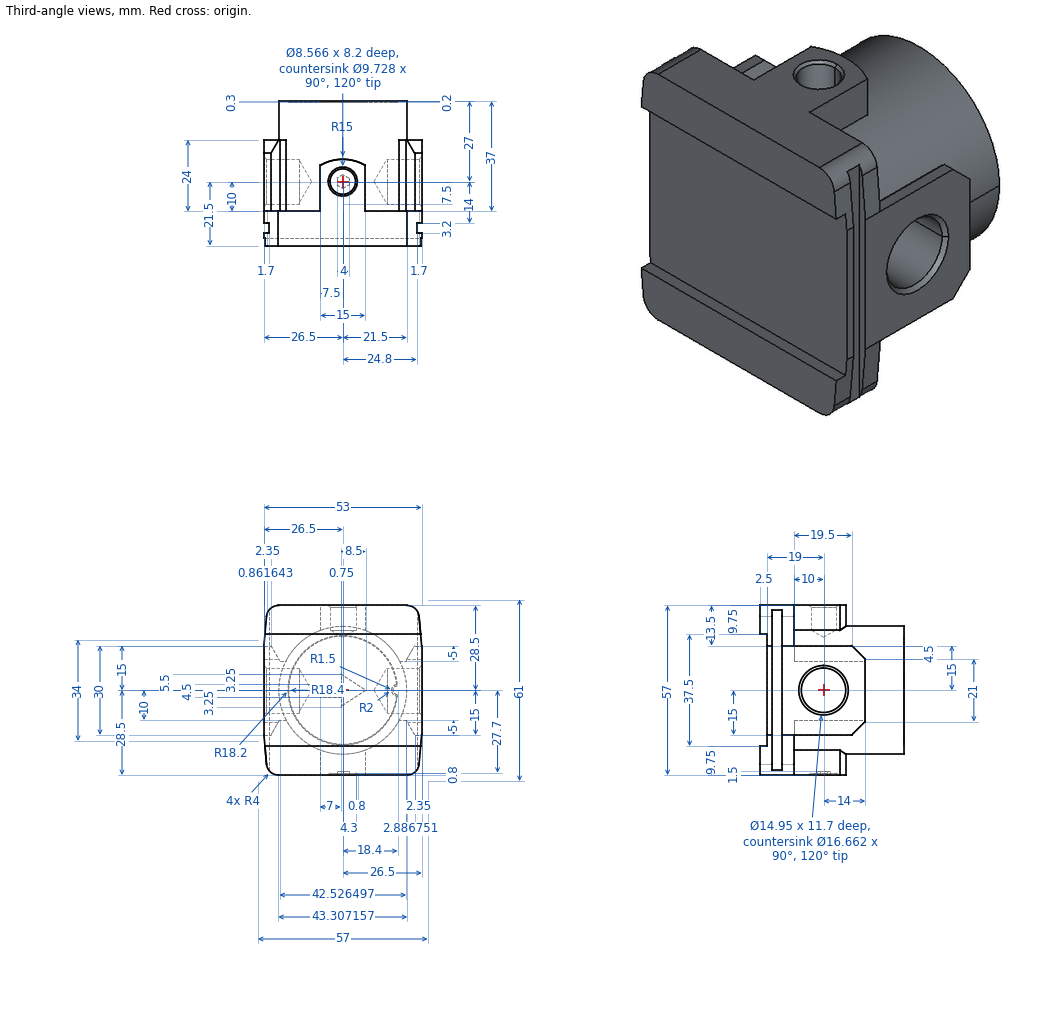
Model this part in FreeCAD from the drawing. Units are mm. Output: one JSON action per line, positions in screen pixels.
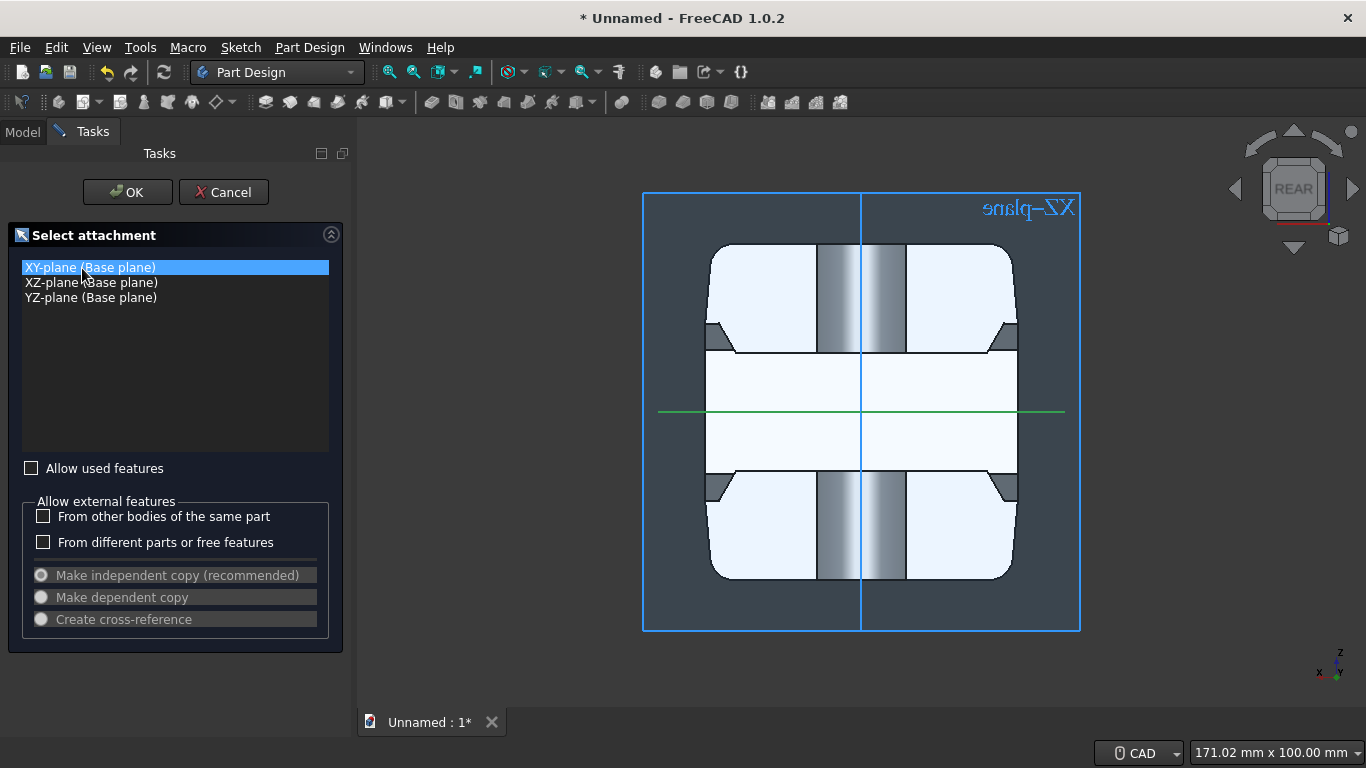
{"action": "left_click", "coordinate": [128, 192]}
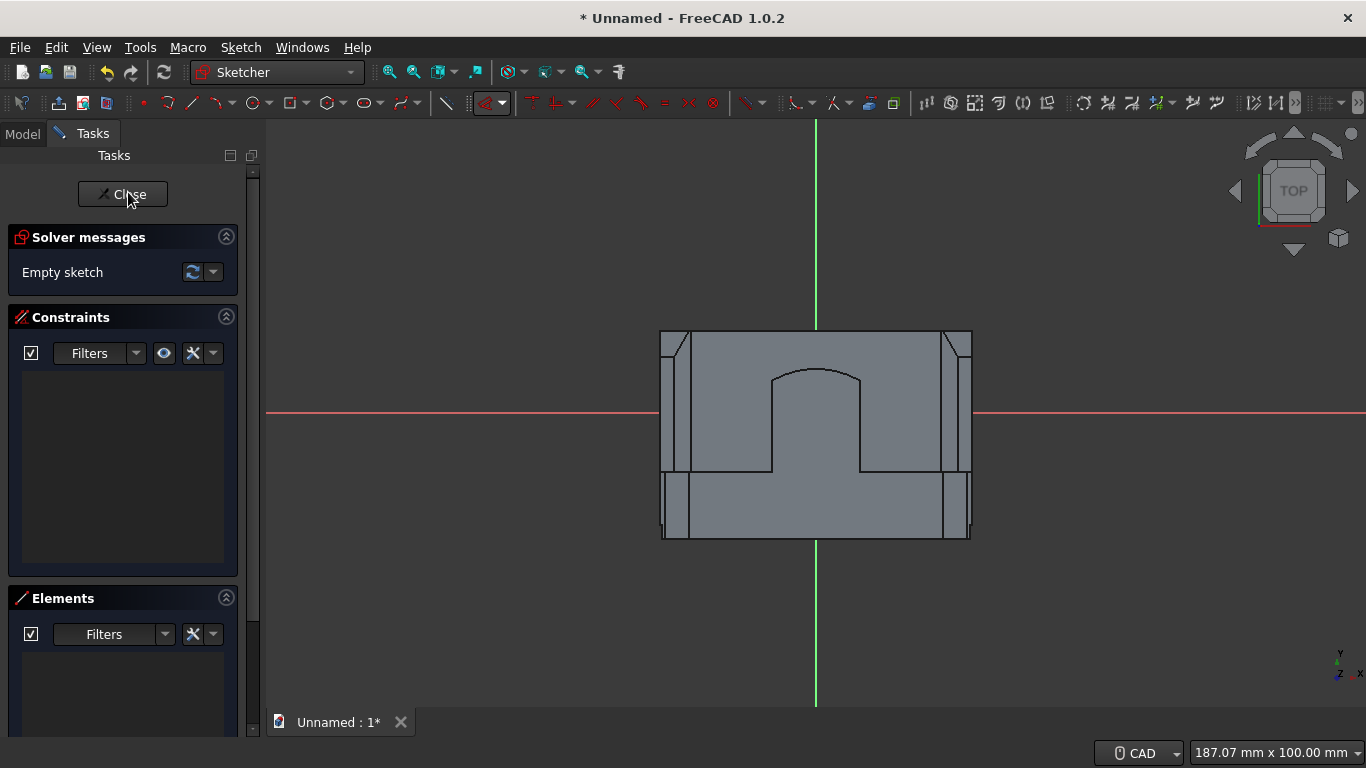
{"action": "left_click", "coordinate": [108, 104]}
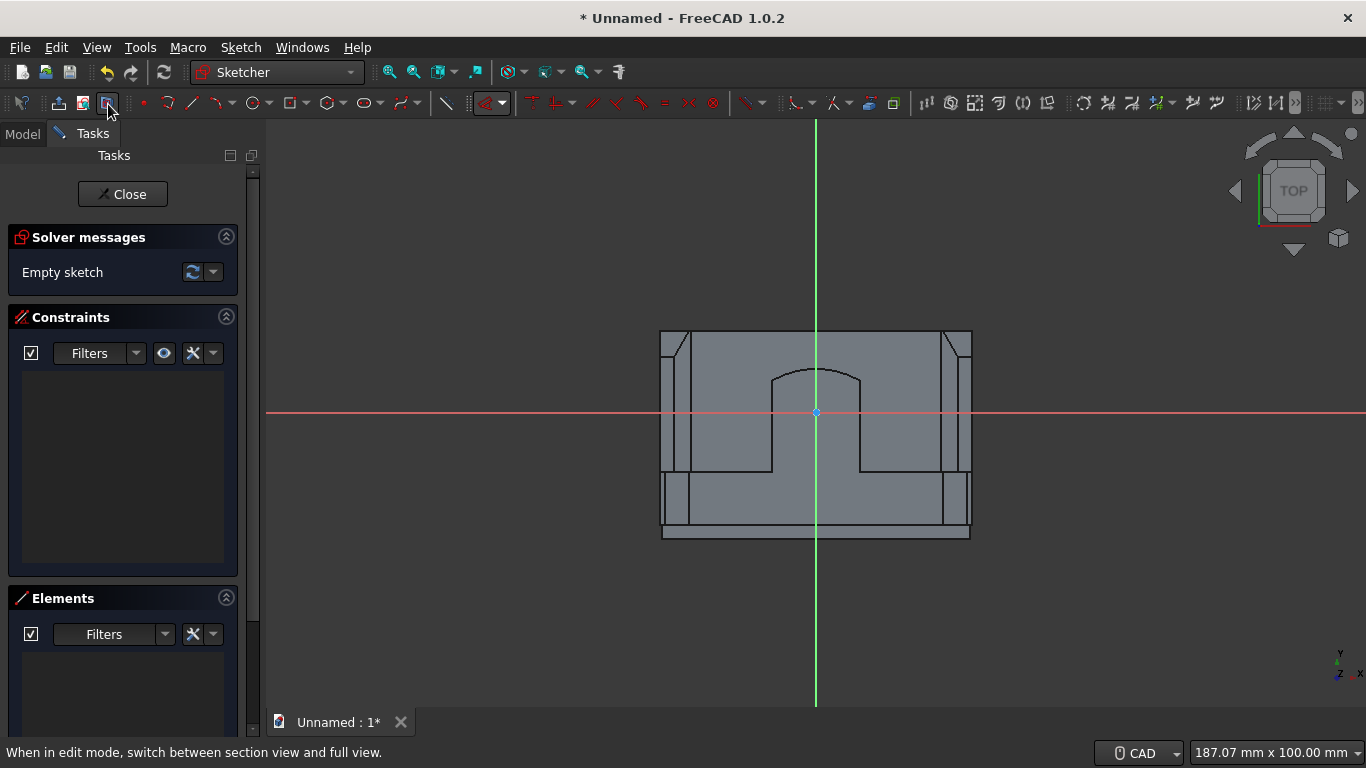
{"action": "scroll", "coordinate": [1039, 302], "scroll_direction": "up", "scroll_amount": 3}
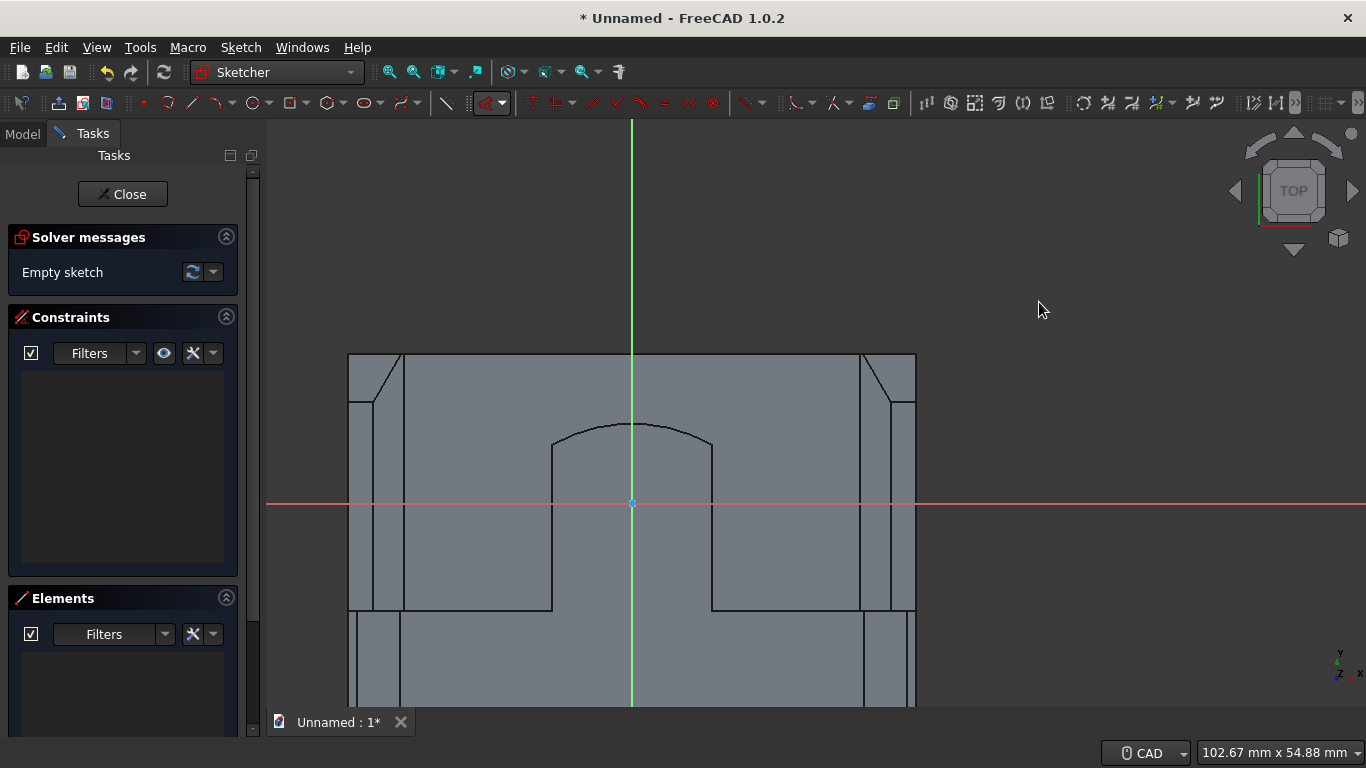
{"action": "key", "text": "g r"}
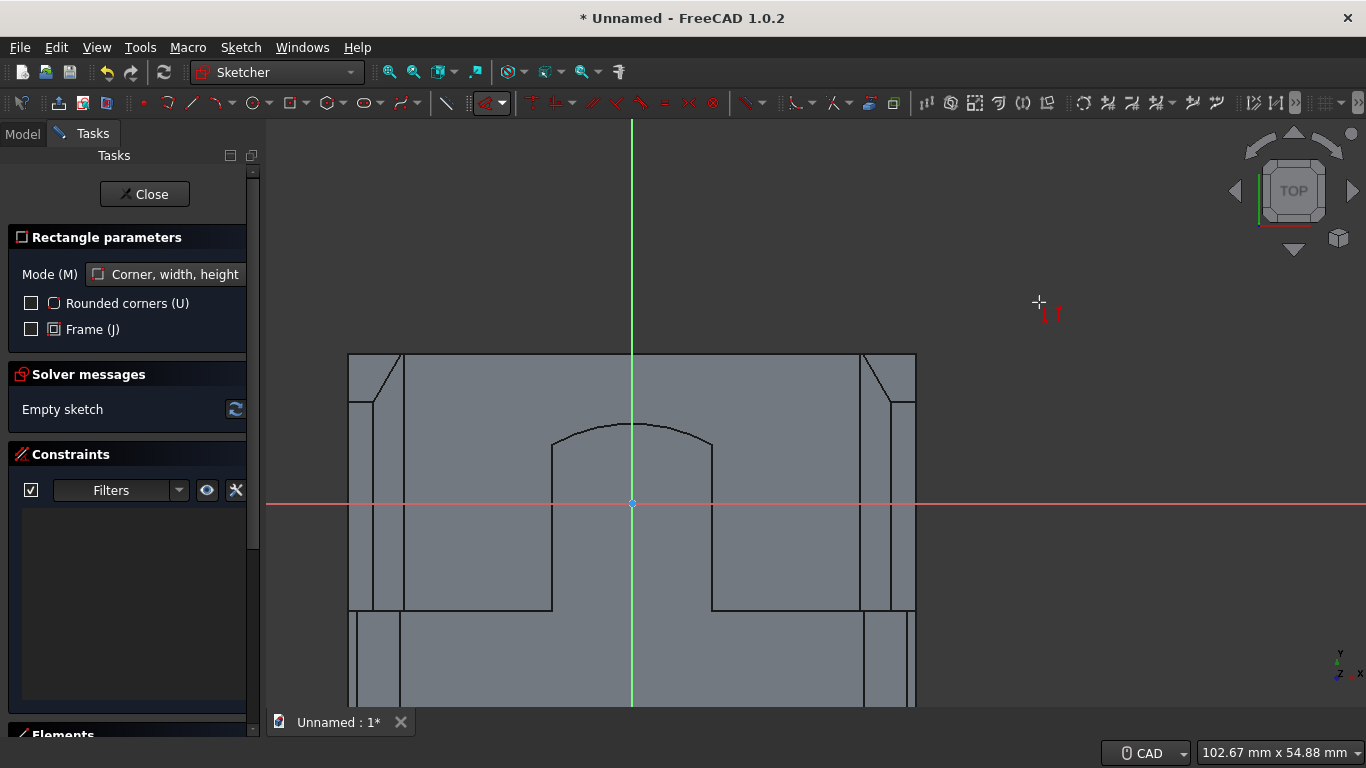
{"action": "left_click", "coordinate": [632, 215]}
{"action": "mouse_move", "coordinate": [862, 611]}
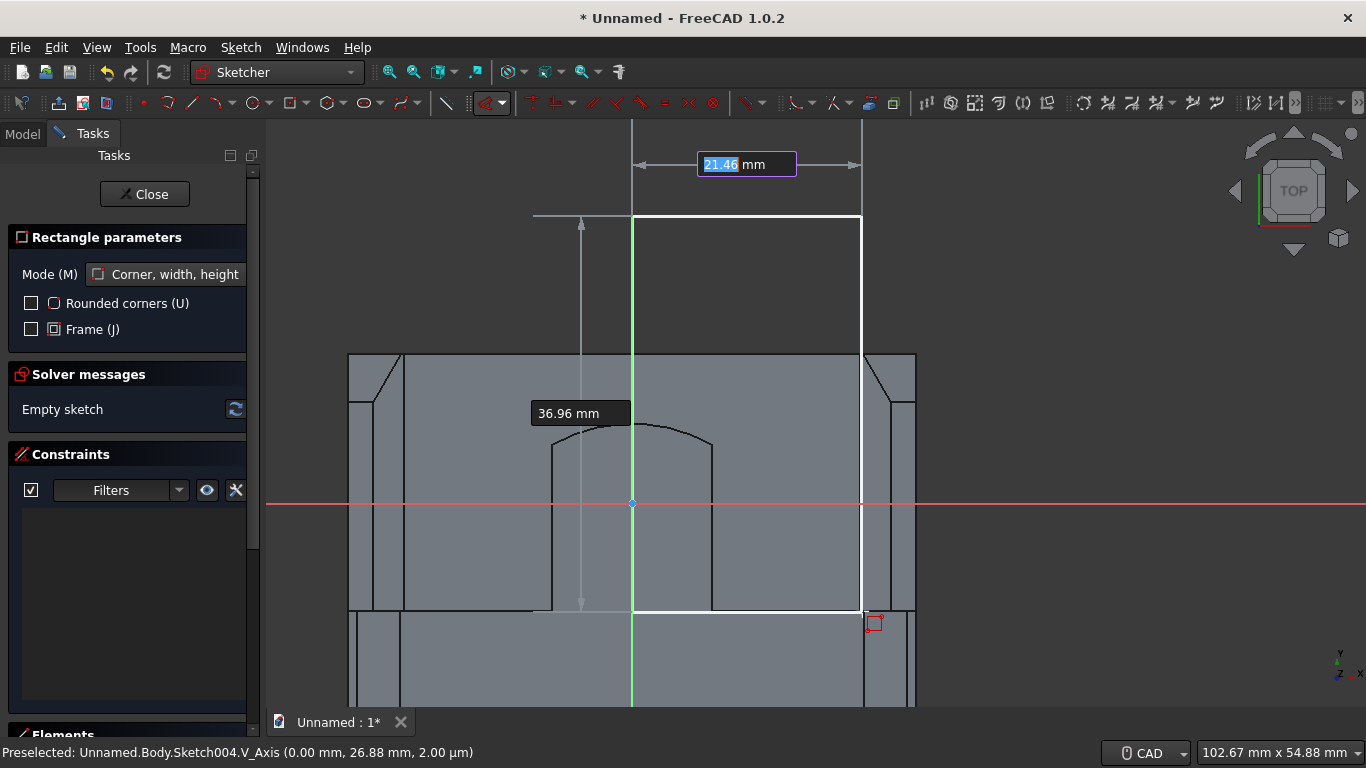
{"action": "type", "text": "21.5"}
{"action": "key", "text": "Tab"}
{"action": "type", "text": "37"}
{"action": "key", "text": "Return"}
{"action": "key", "text": "Escape"}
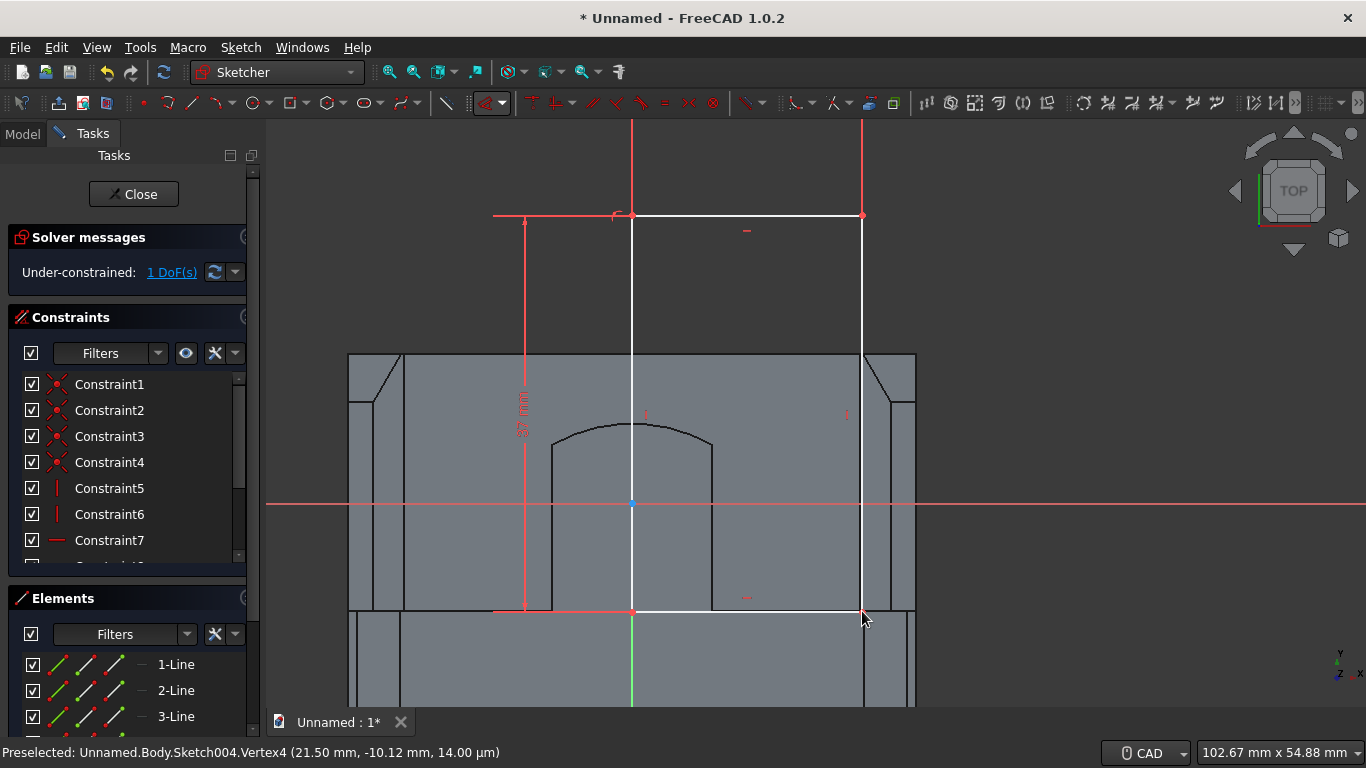
{"action": "left_click", "coordinate": [632, 216]}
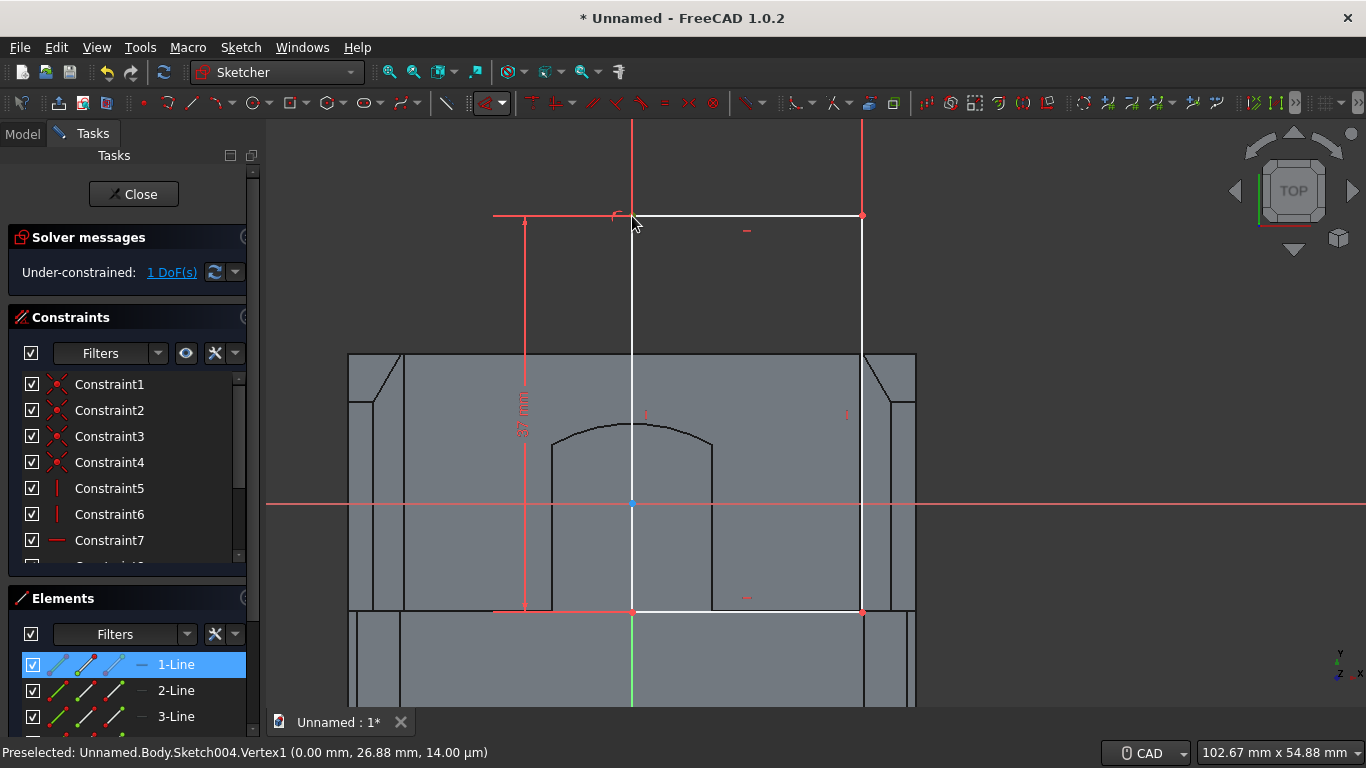
{"action": "left_click", "coordinate": [504, 104]}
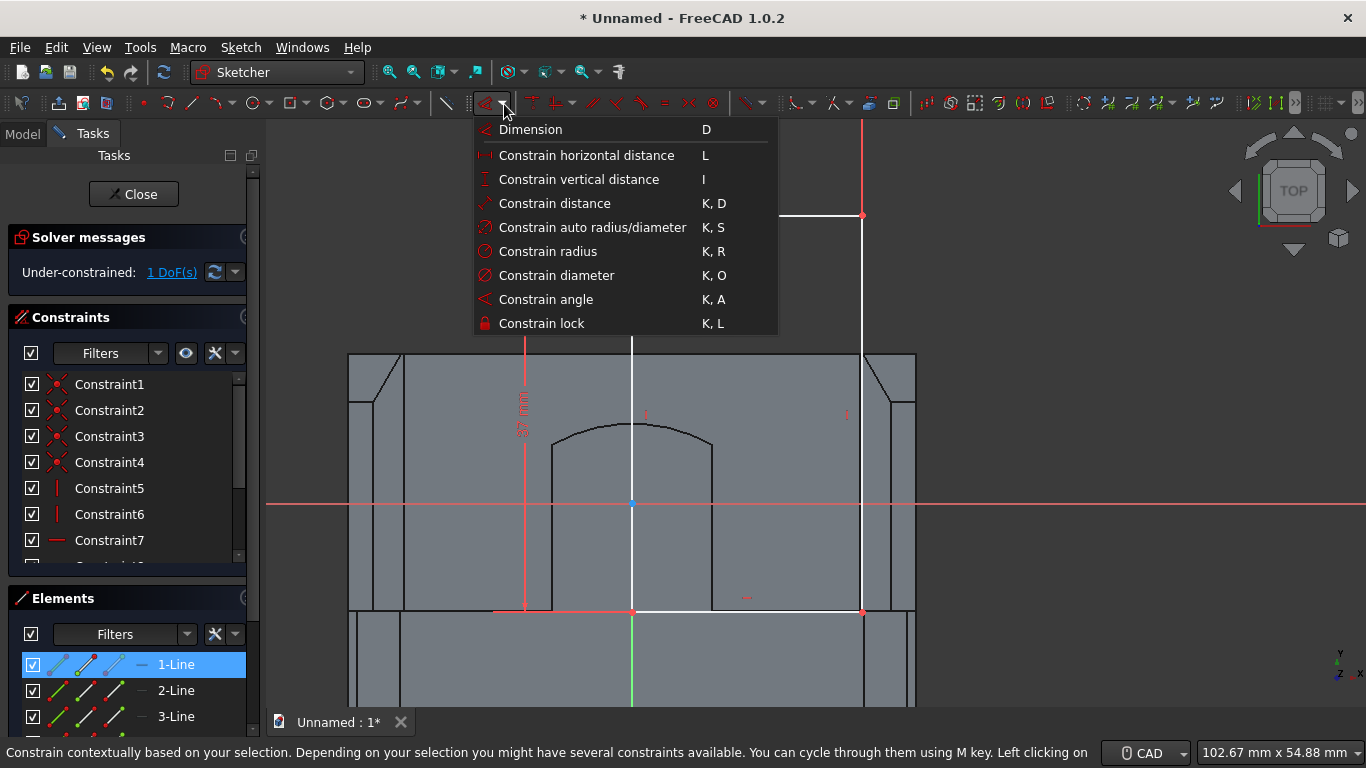
{"action": "left_click", "coordinate": [626, 179]}